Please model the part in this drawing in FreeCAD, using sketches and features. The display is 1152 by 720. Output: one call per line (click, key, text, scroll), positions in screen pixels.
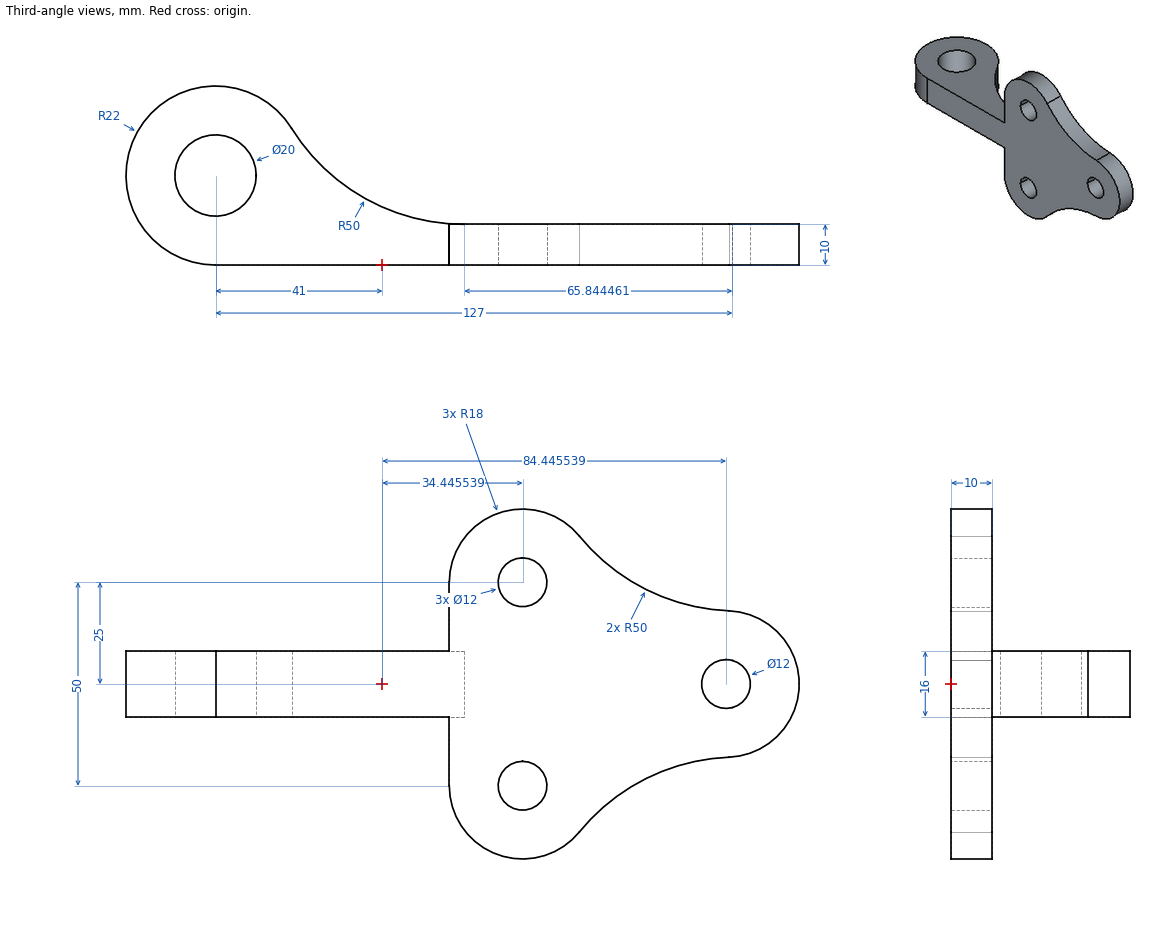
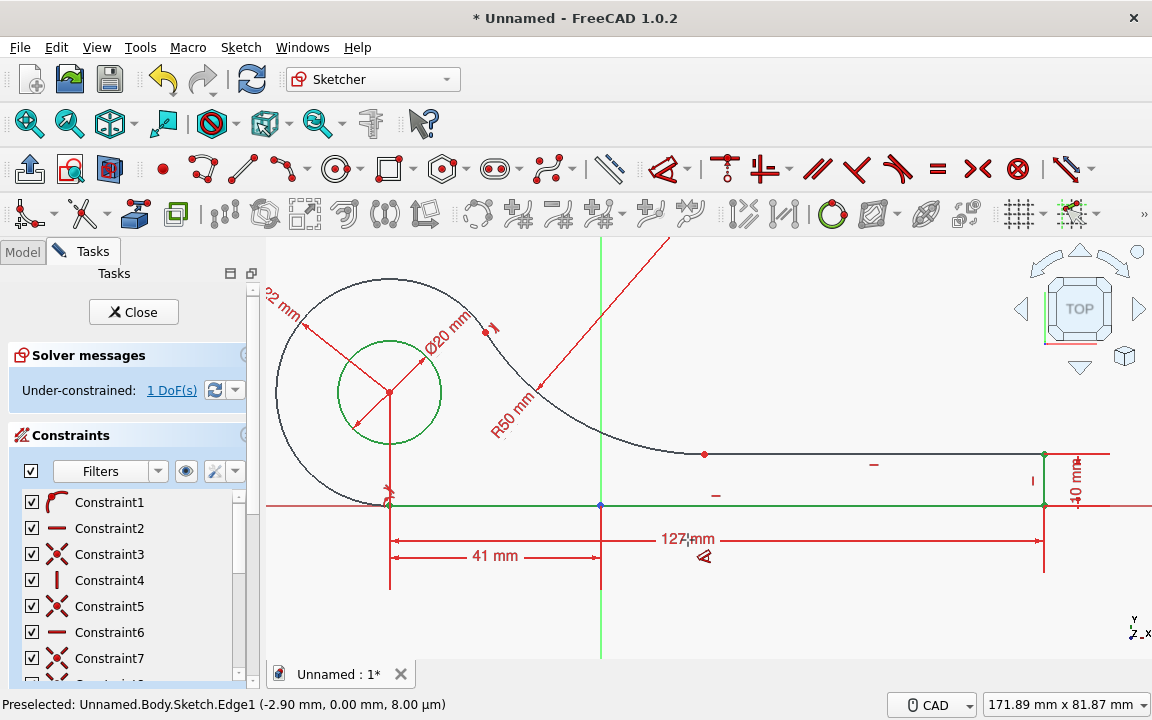
click(942, 454)
click(846, 488)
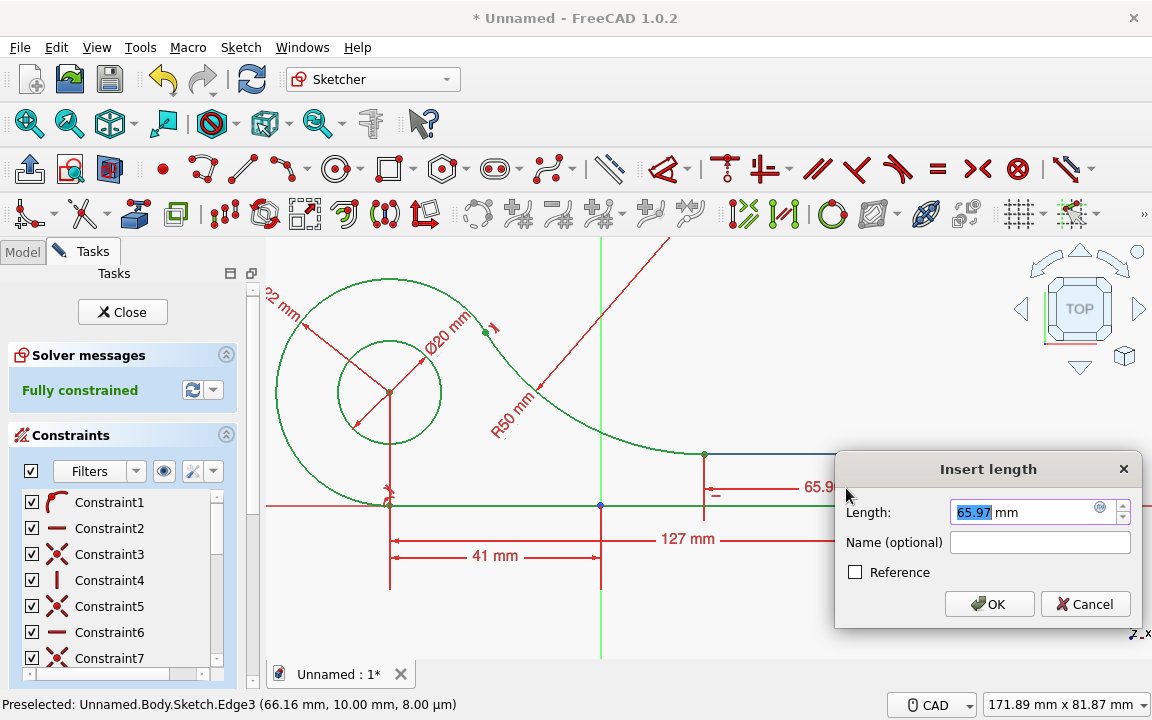
text(65.844461)
key(Return)
key(Escape)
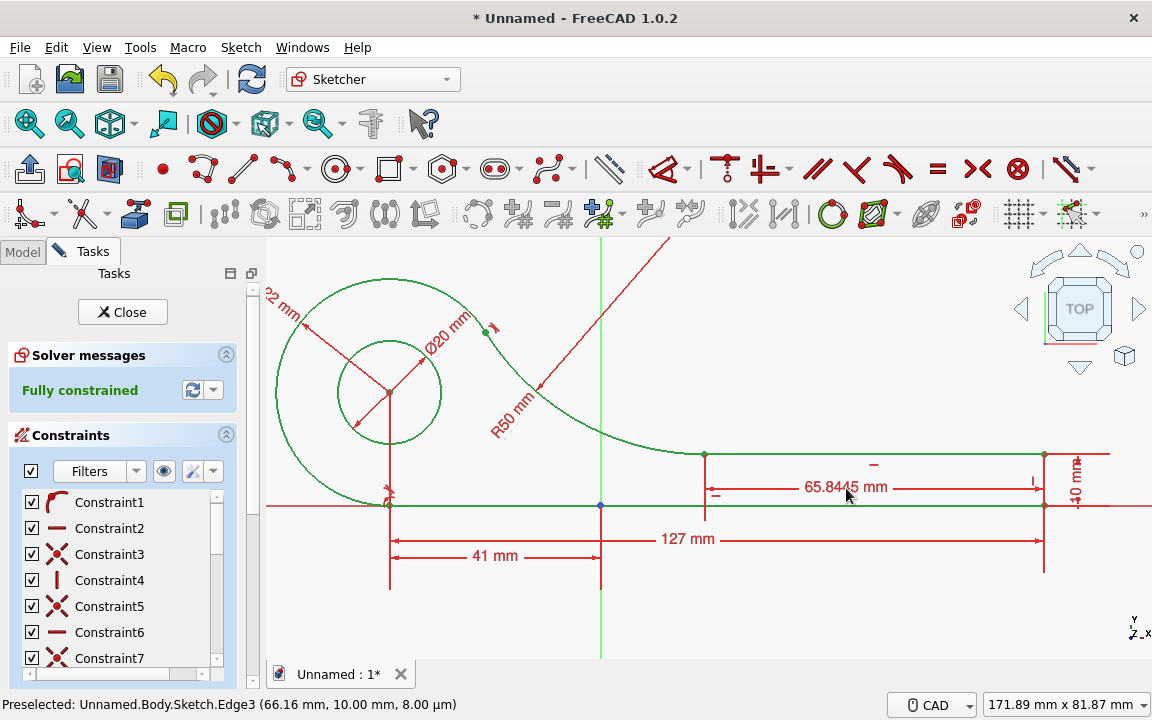
click(123, 312)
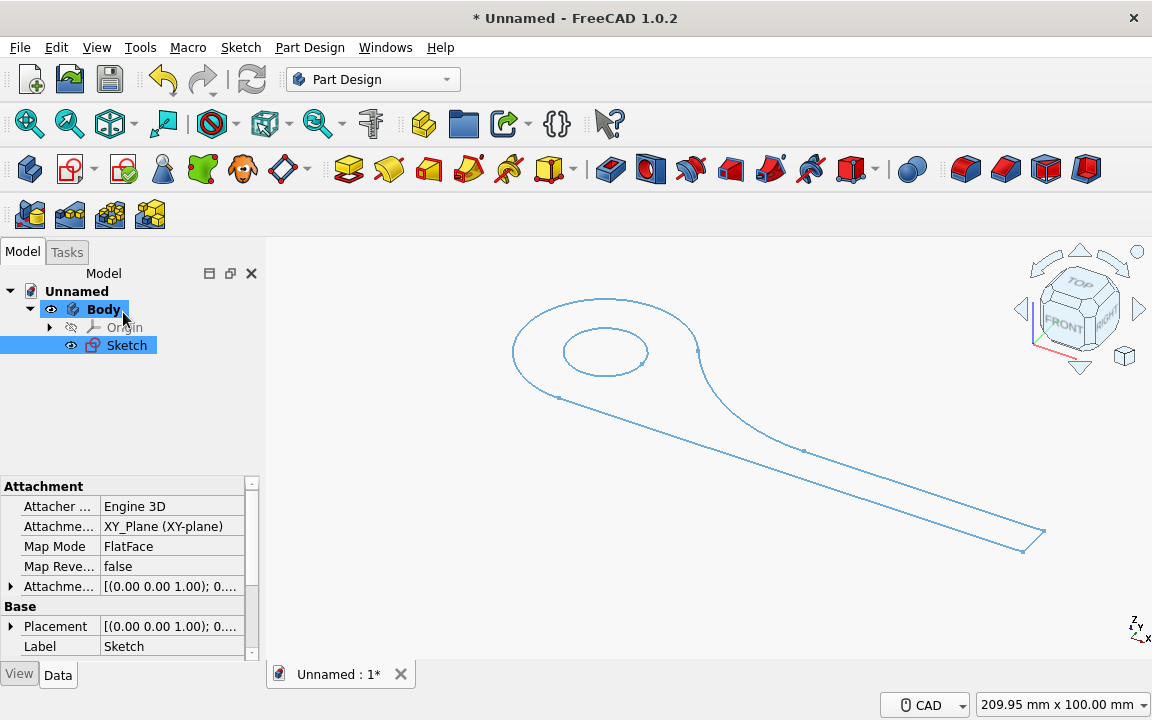
click(350, 170)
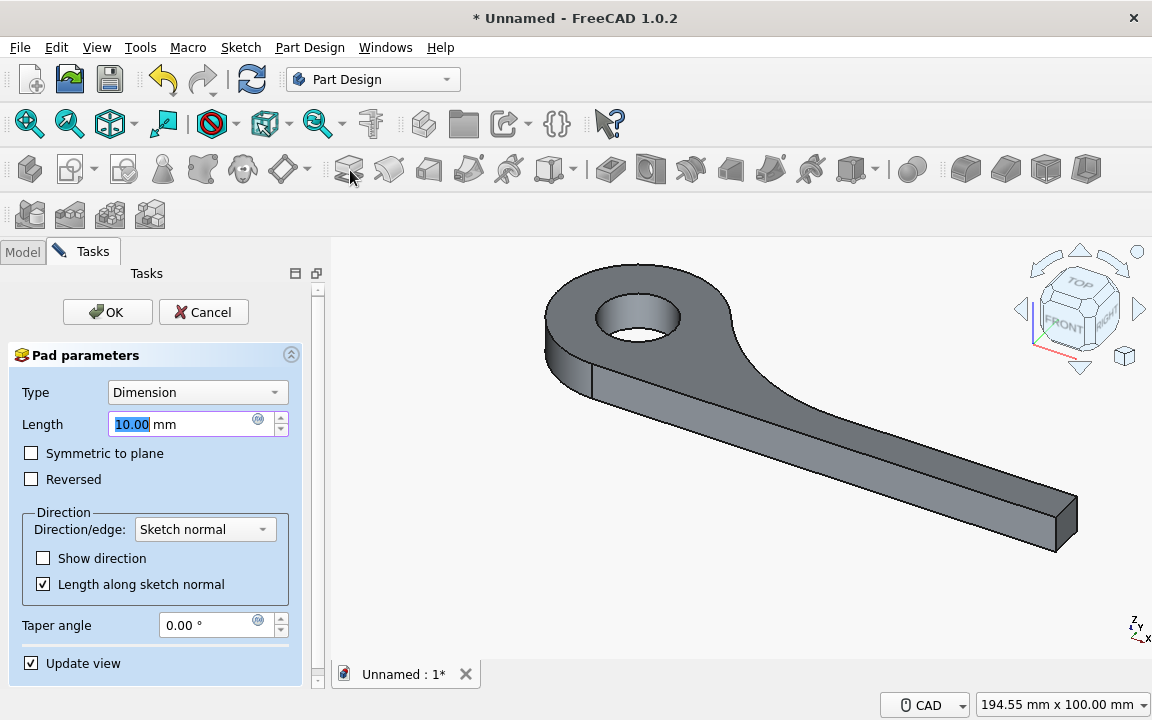
text(16)
key(Tab)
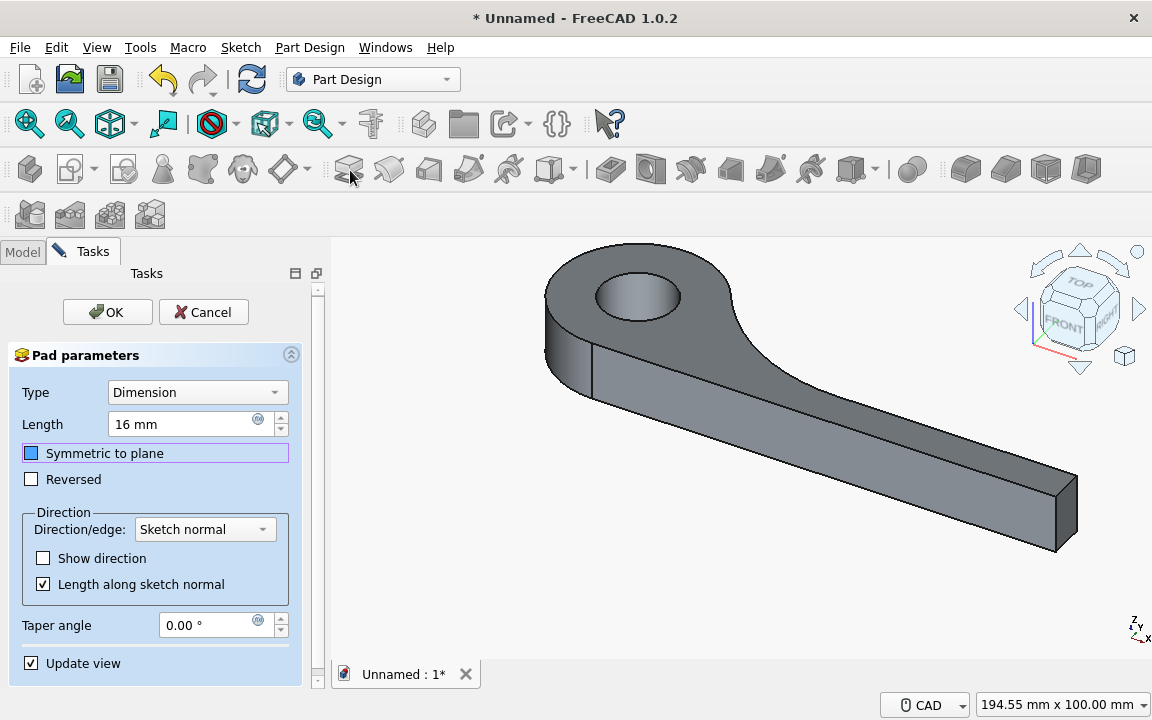
click(30, 453)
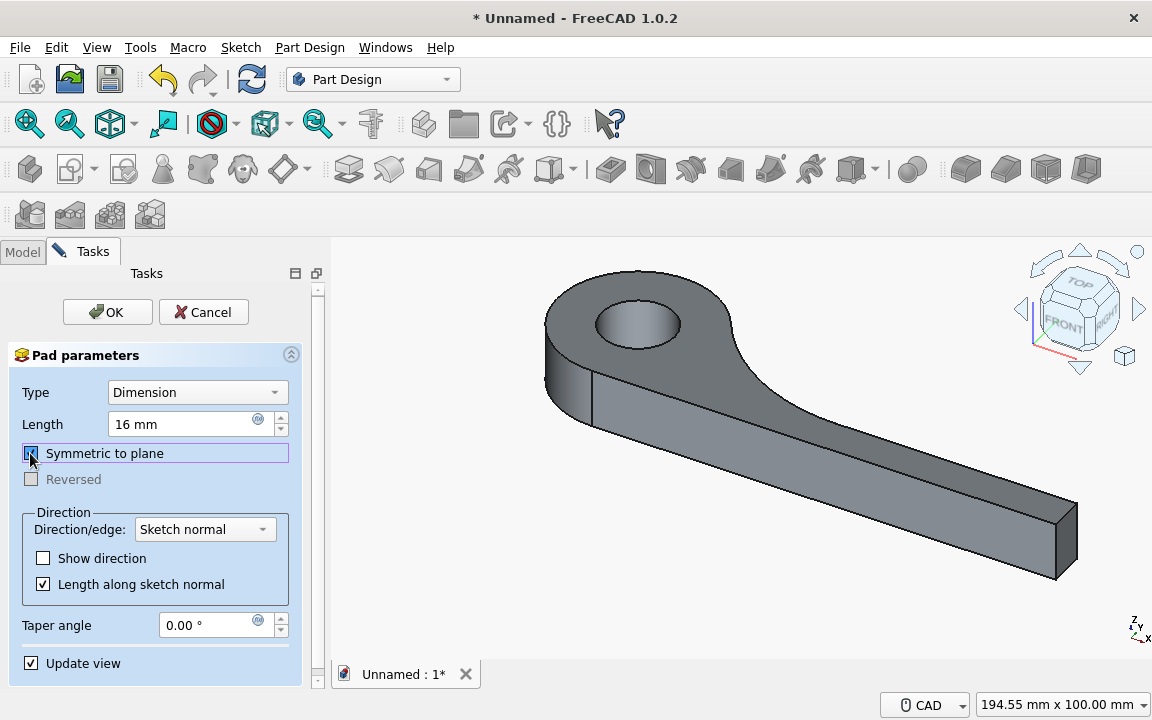
click(108, 312)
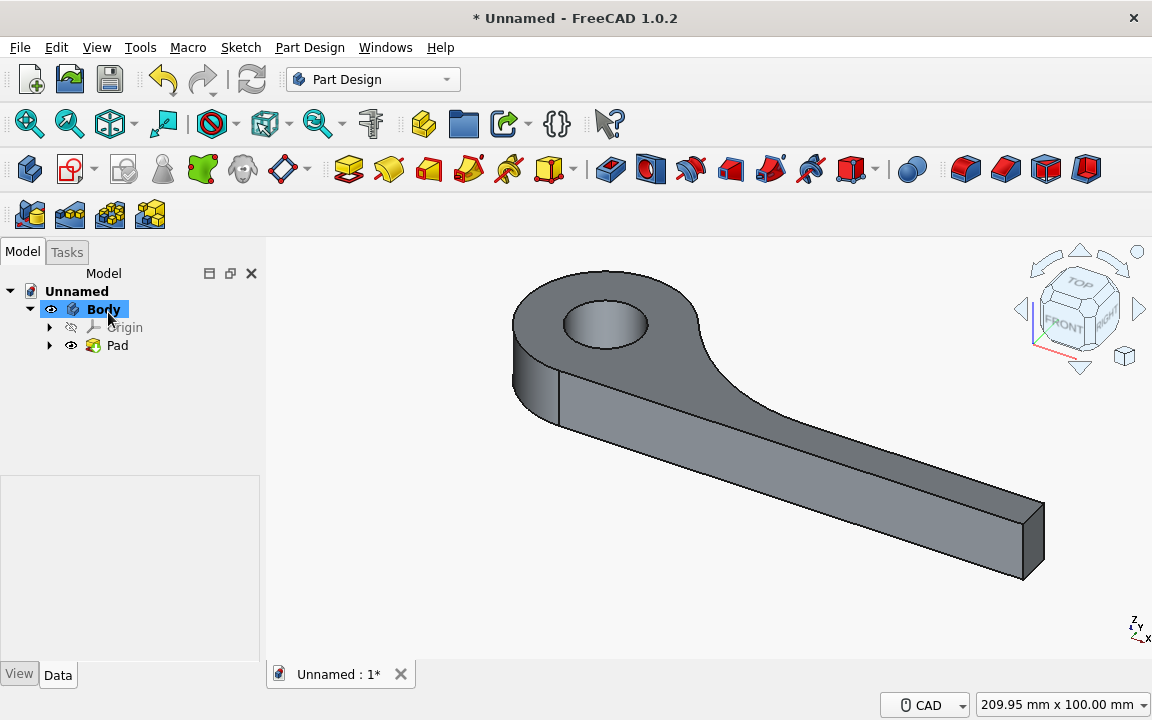
key(4)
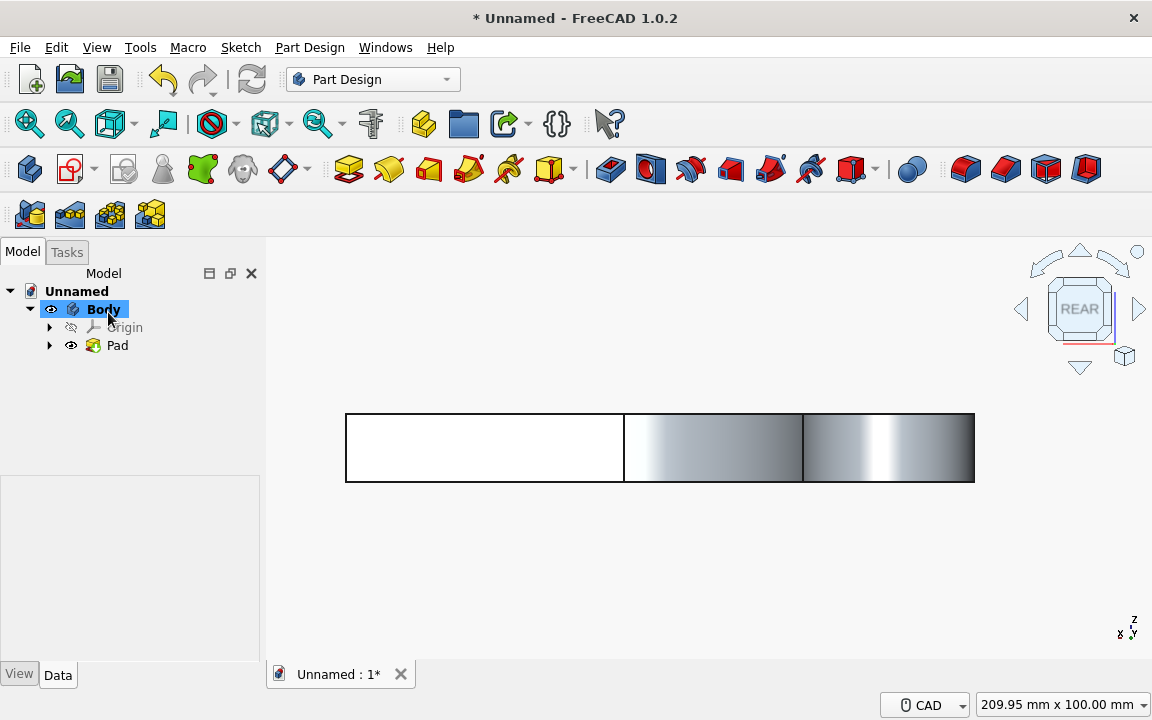
click(406, 447)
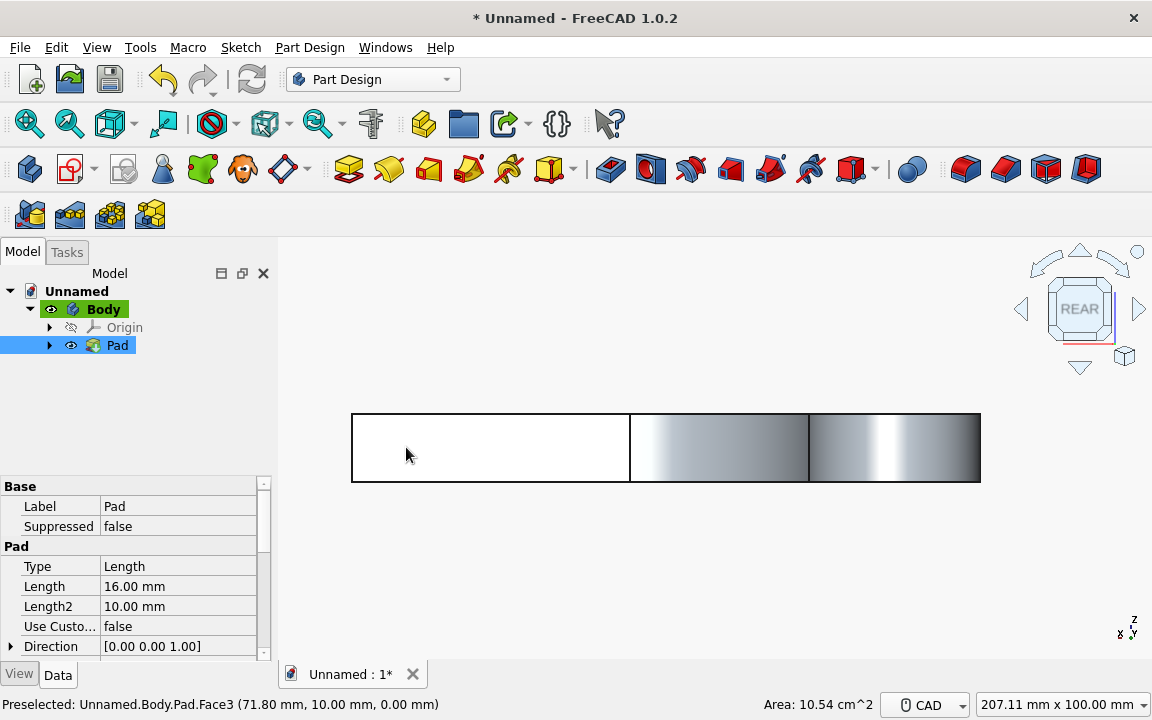
click(70, 170)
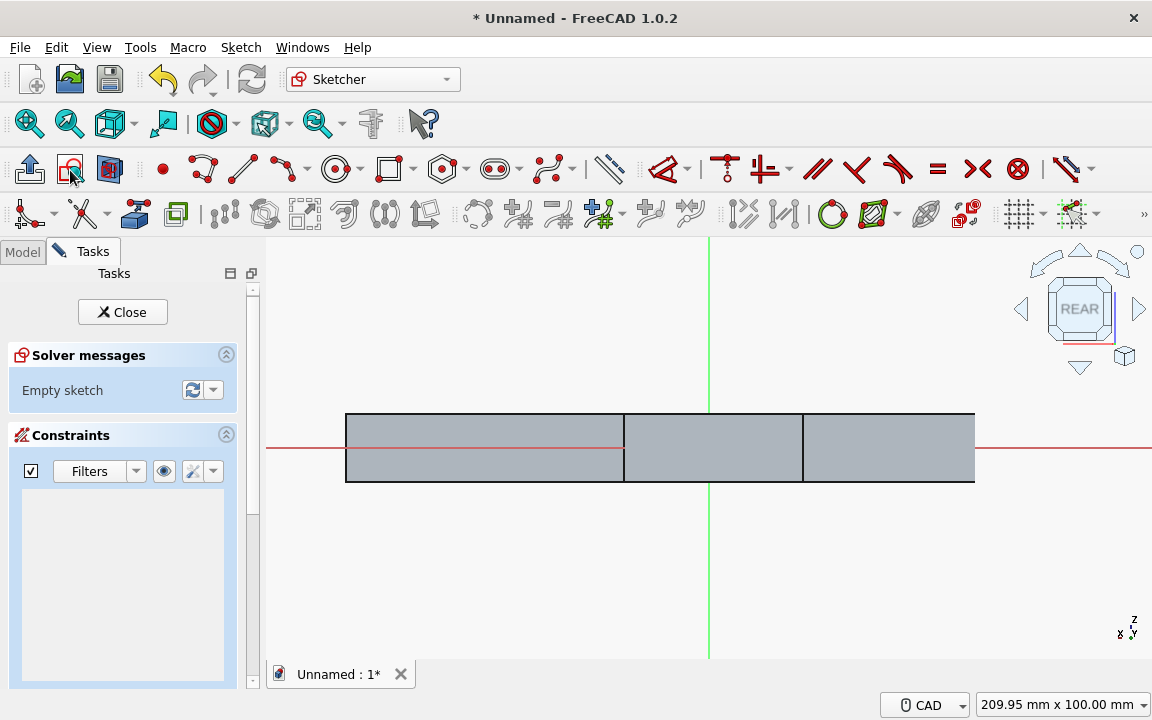
scroll(941, 448, down, 2)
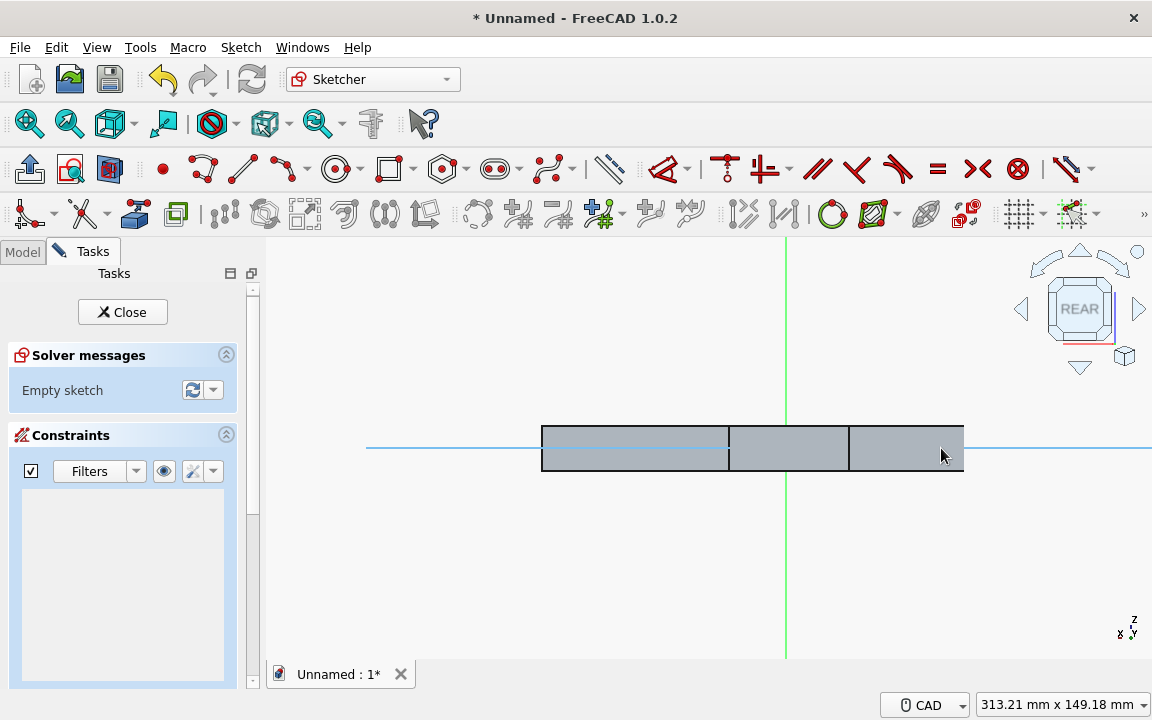
key(g)
key(l)